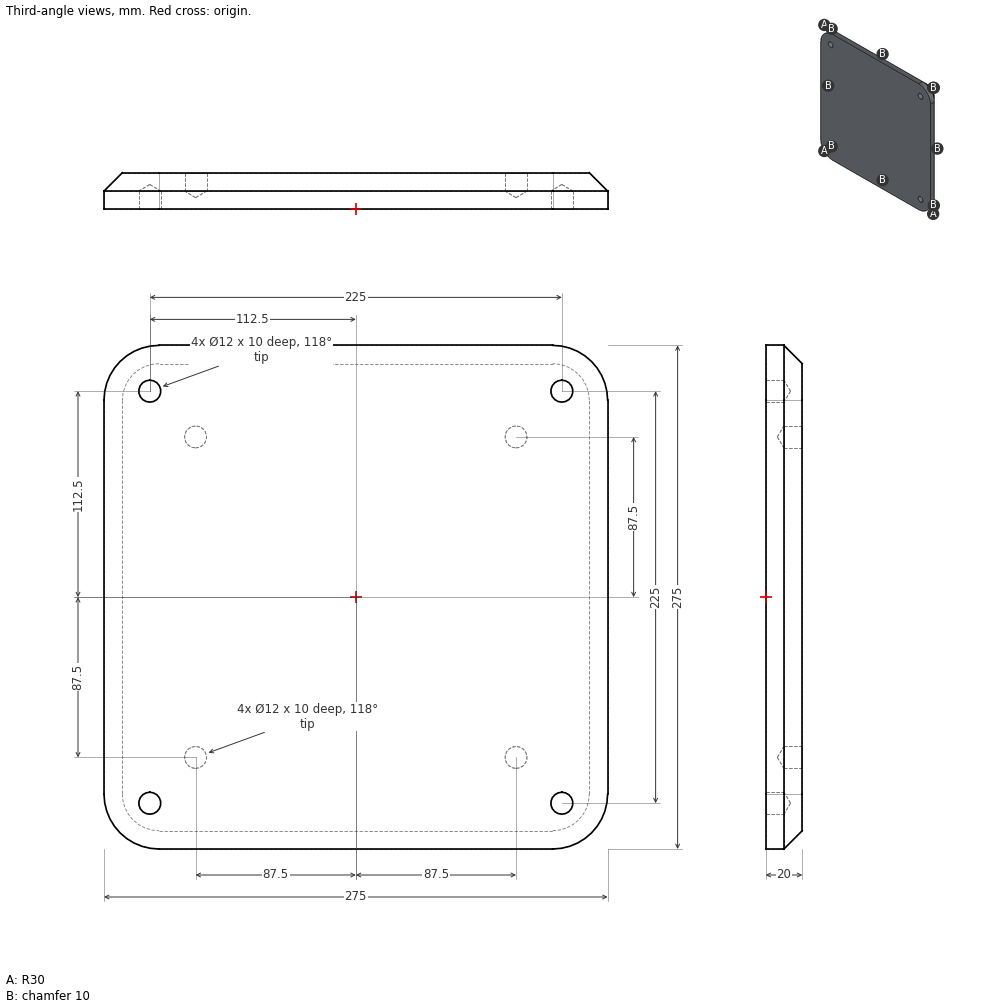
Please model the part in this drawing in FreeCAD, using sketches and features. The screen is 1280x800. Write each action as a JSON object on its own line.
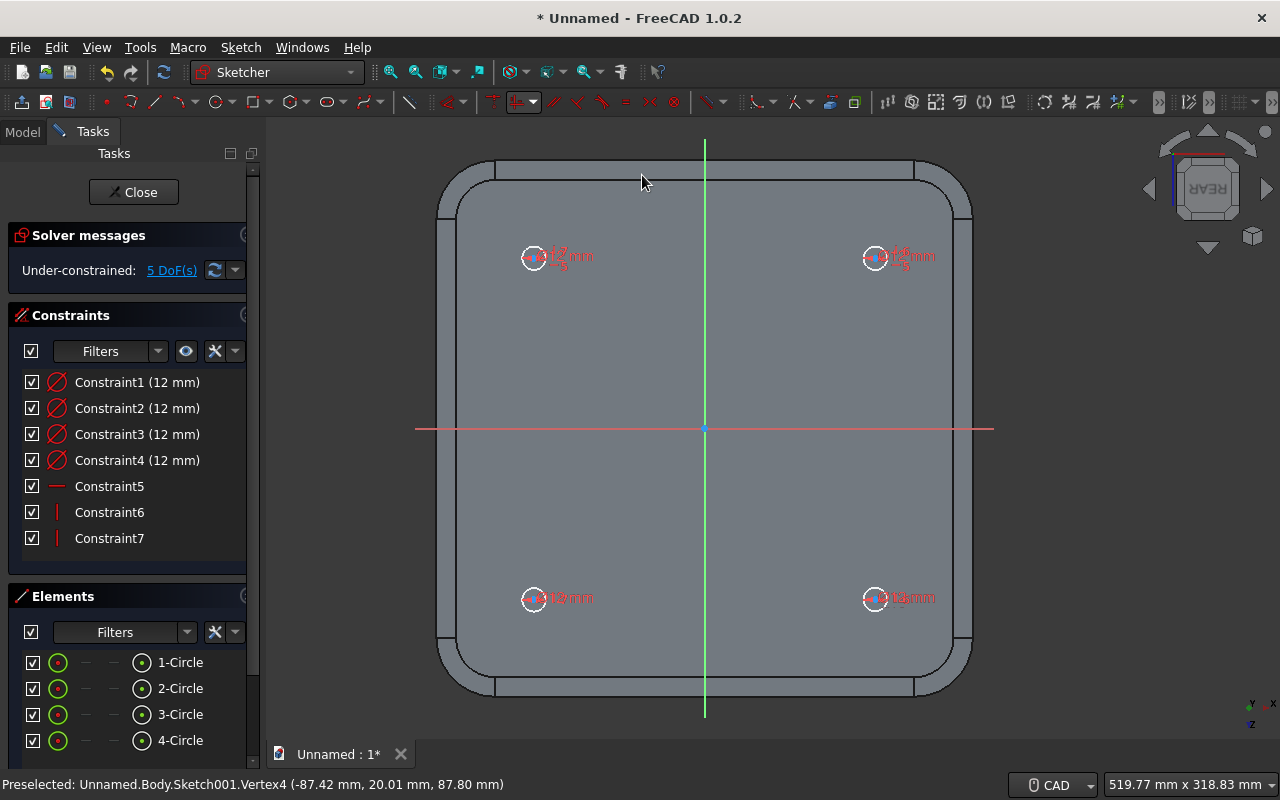
{"action": "left_click", "coordinate": [875, 600]}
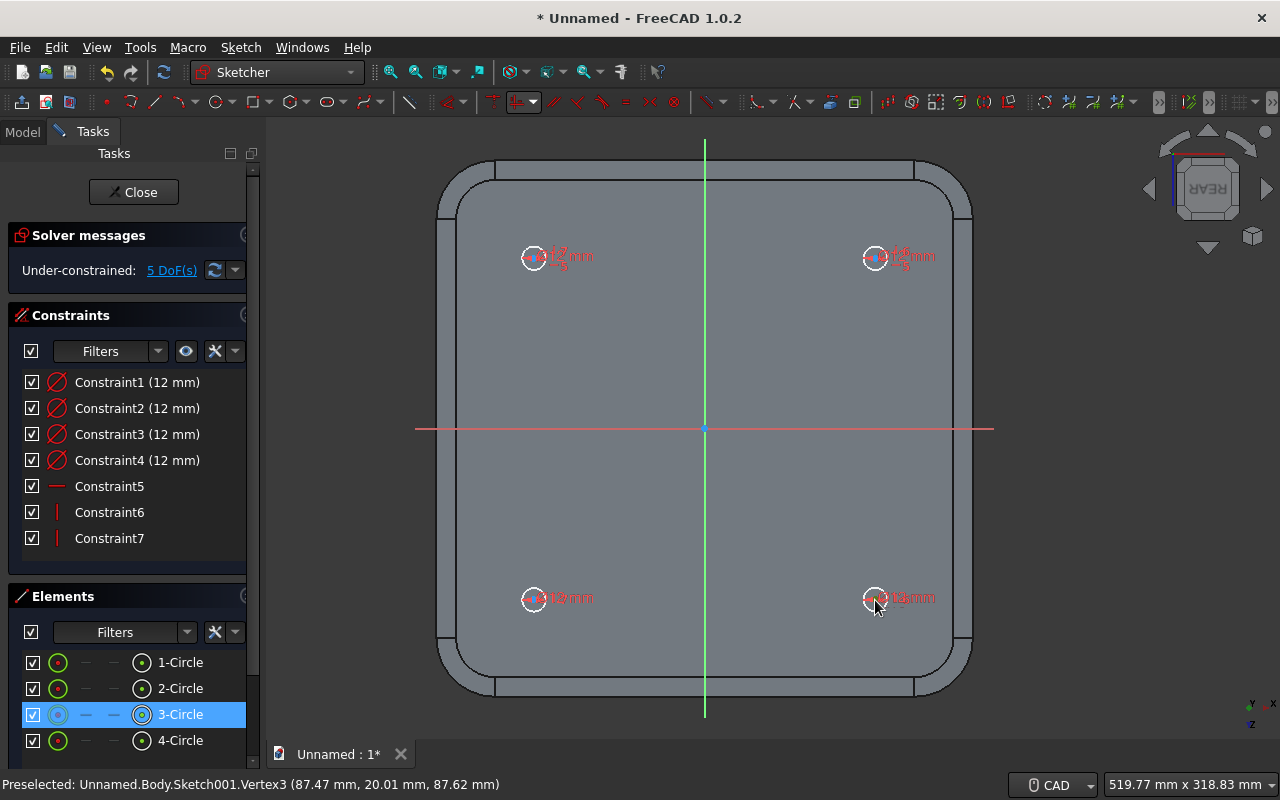
{"action": "left_click", "coordinate": [534, 600]}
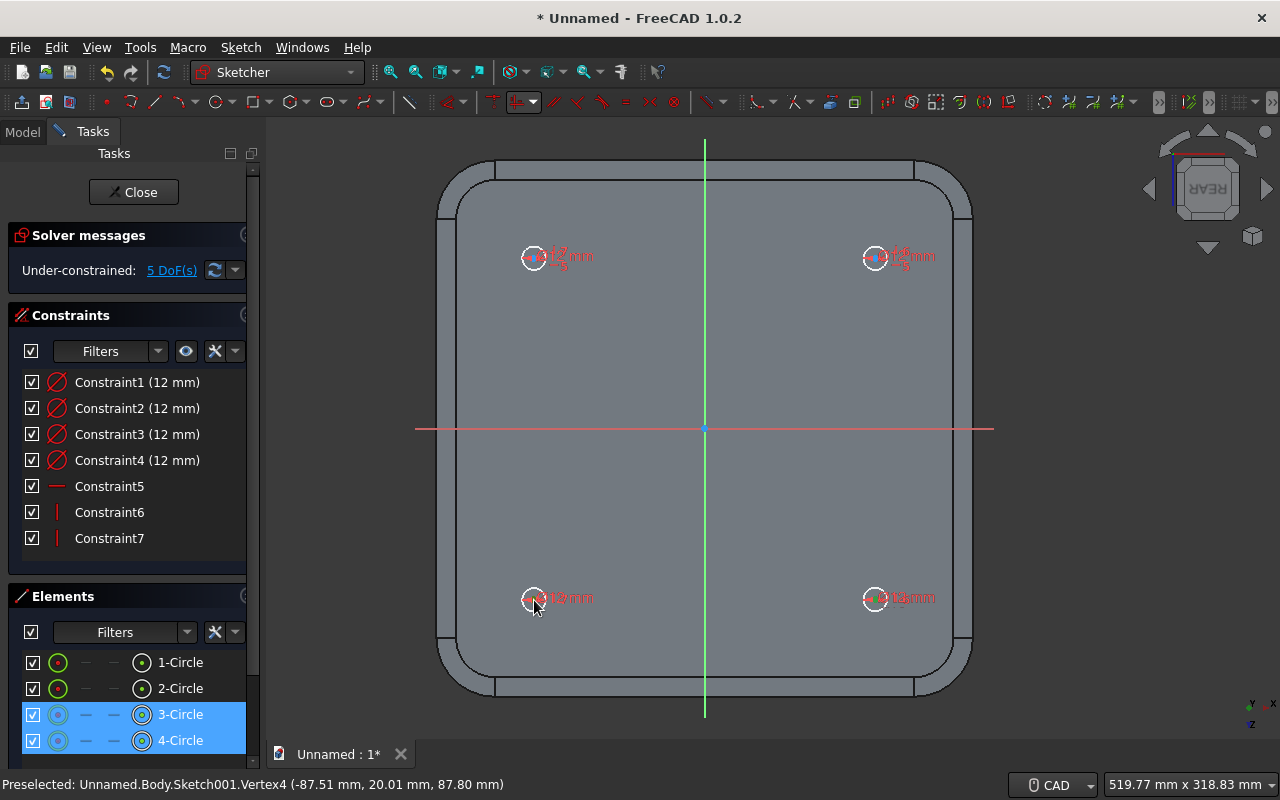
{"action": "key", "text": "h"}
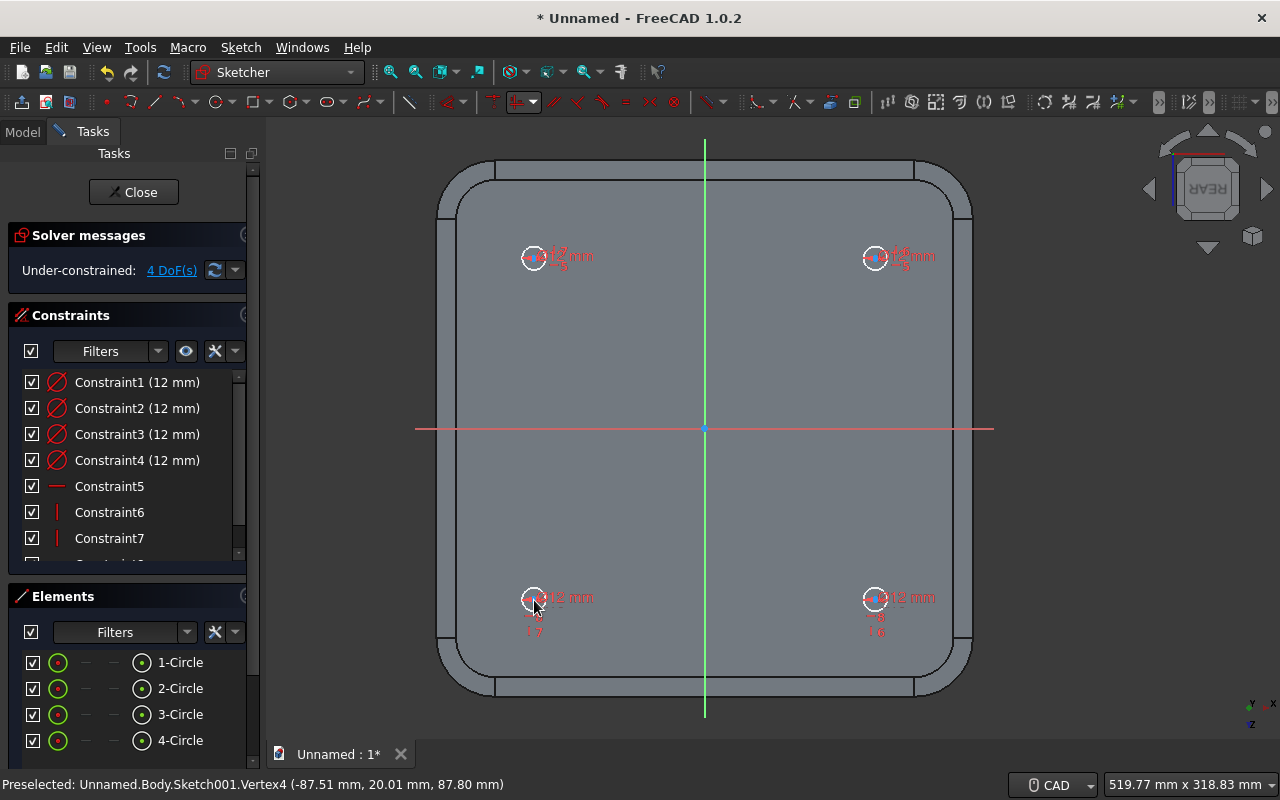
{"action": "key", "text": "d"}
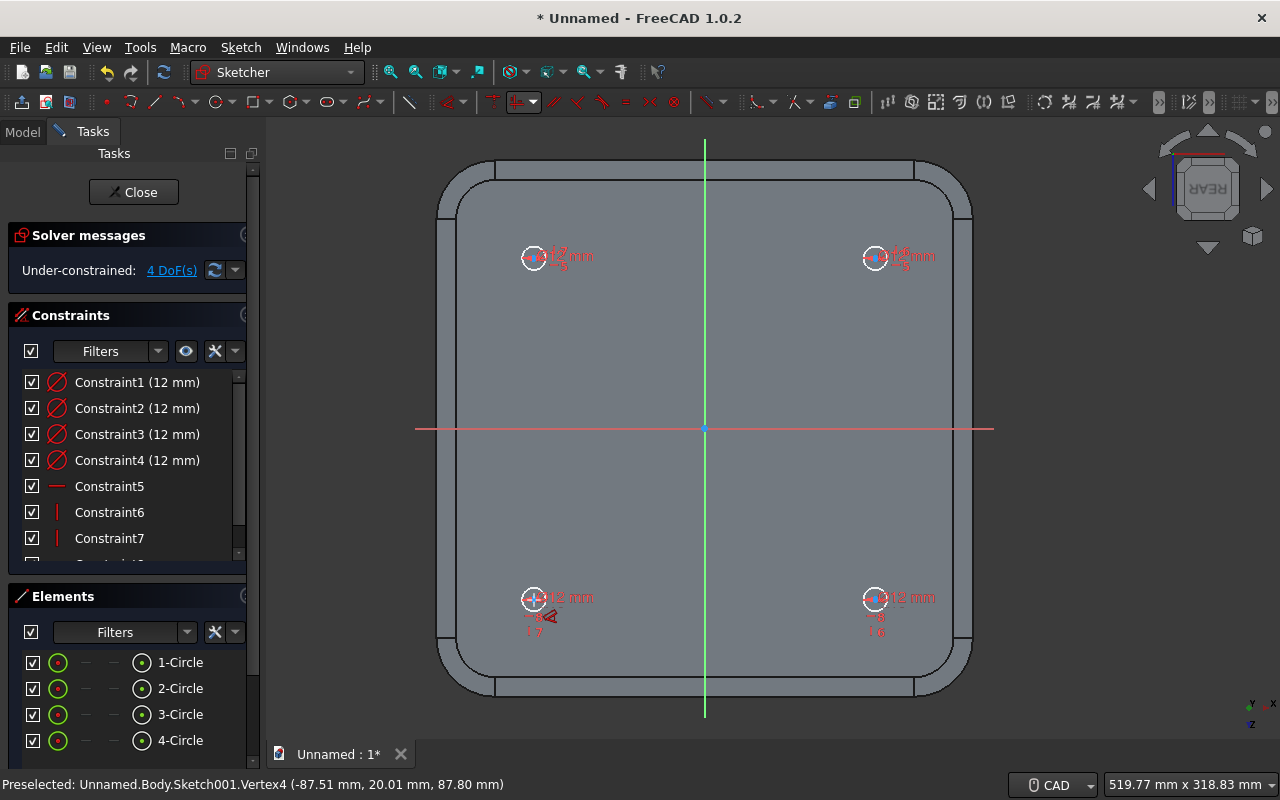
{"action": "left_click", "coordinate": [534, 258]}
{"action": "left_click", "coordinate": [619, 224]}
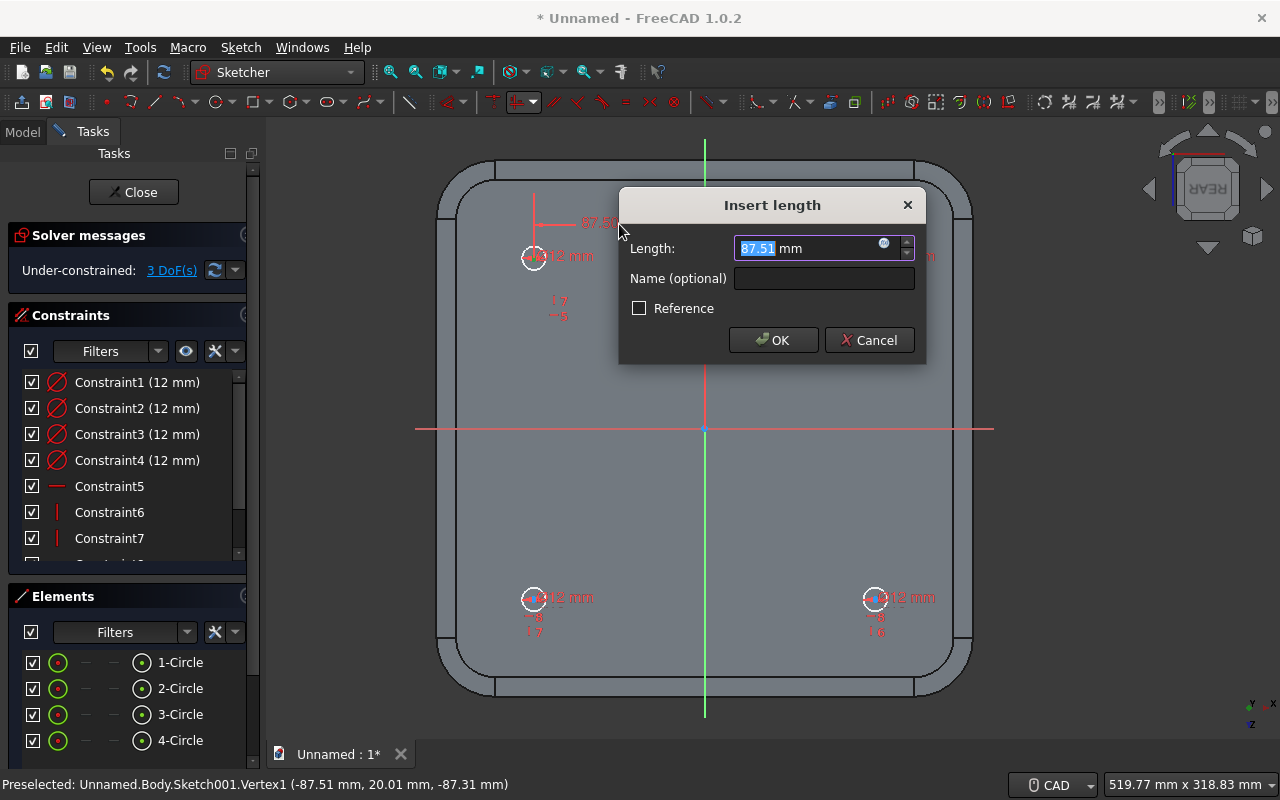
{"action": "type", "text": "87.5"}
{"action": "key", "text": "Return"}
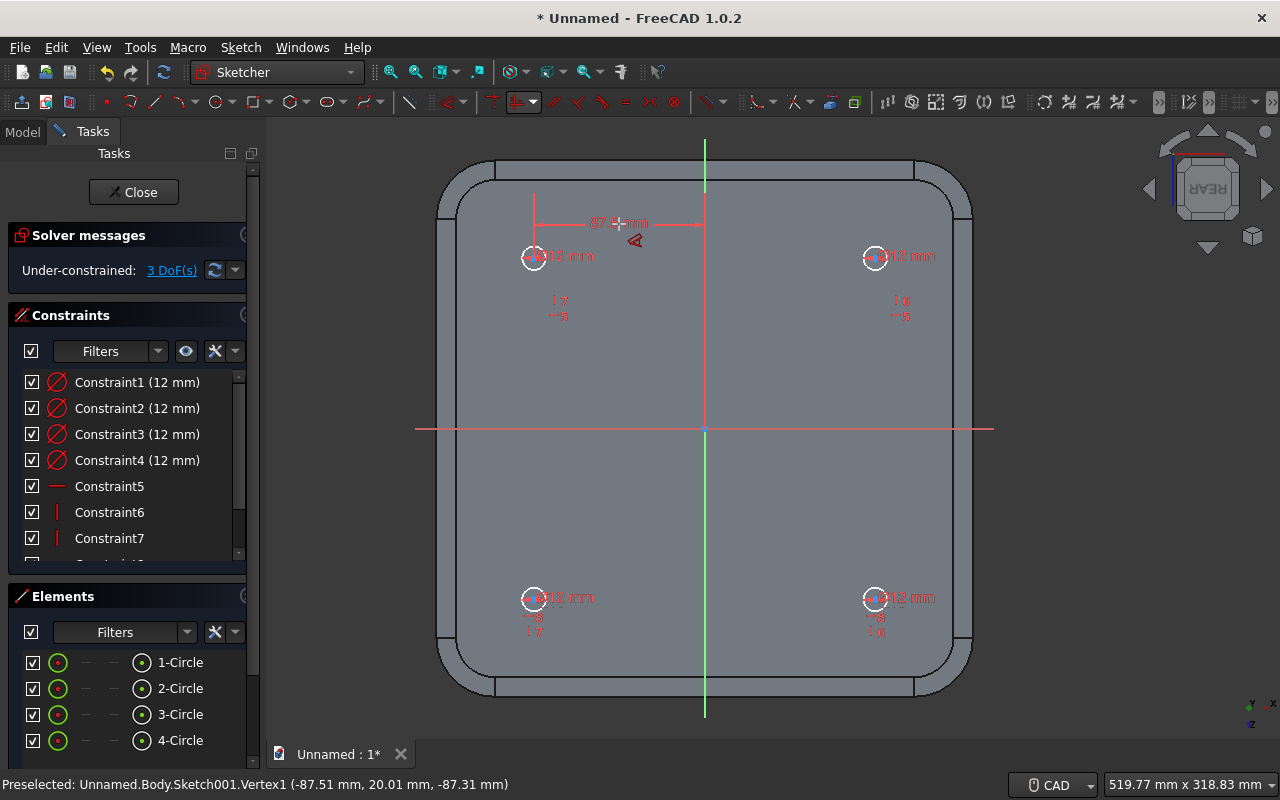
{"action": "left_click", "coordinate": [534, 258]}
{"action": "left_click", "coordinate": [500, 343]}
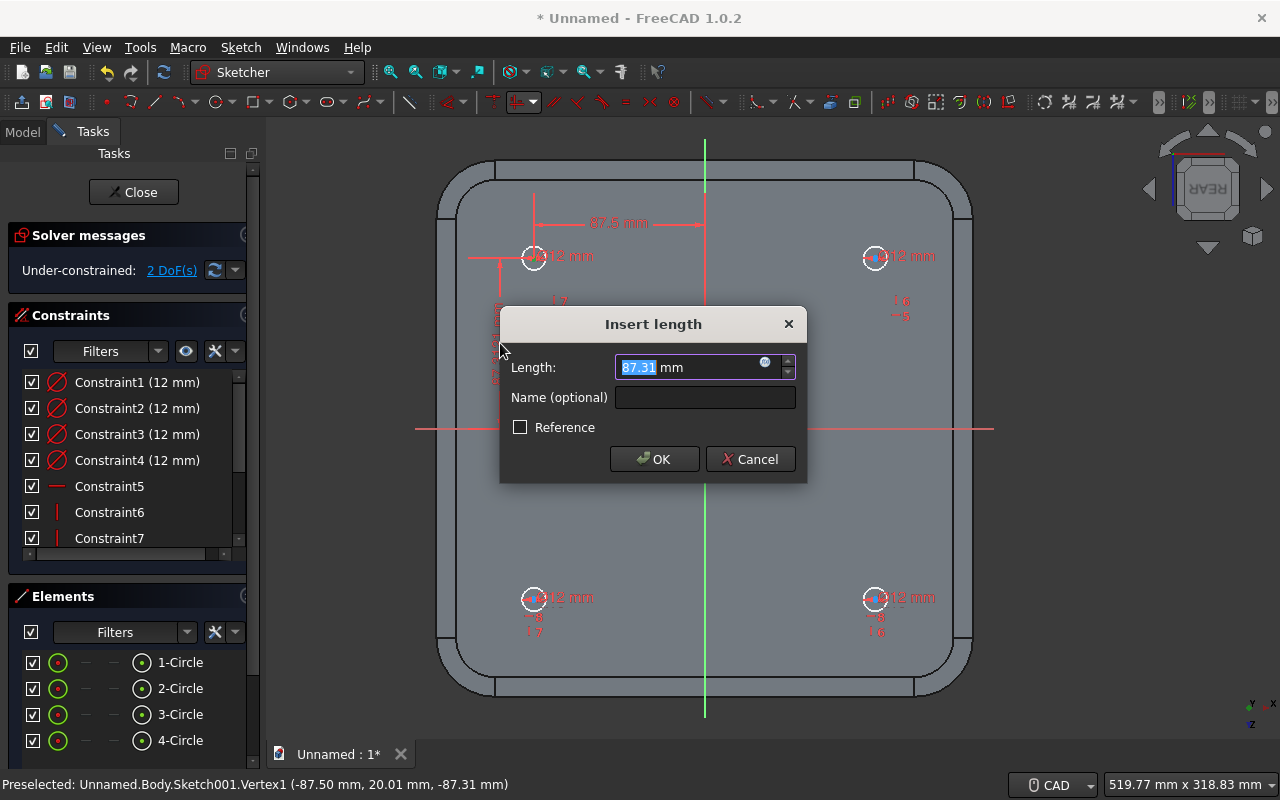
{"action": "type", "text": "87.5"}
{"action": "key", "text": "Return"}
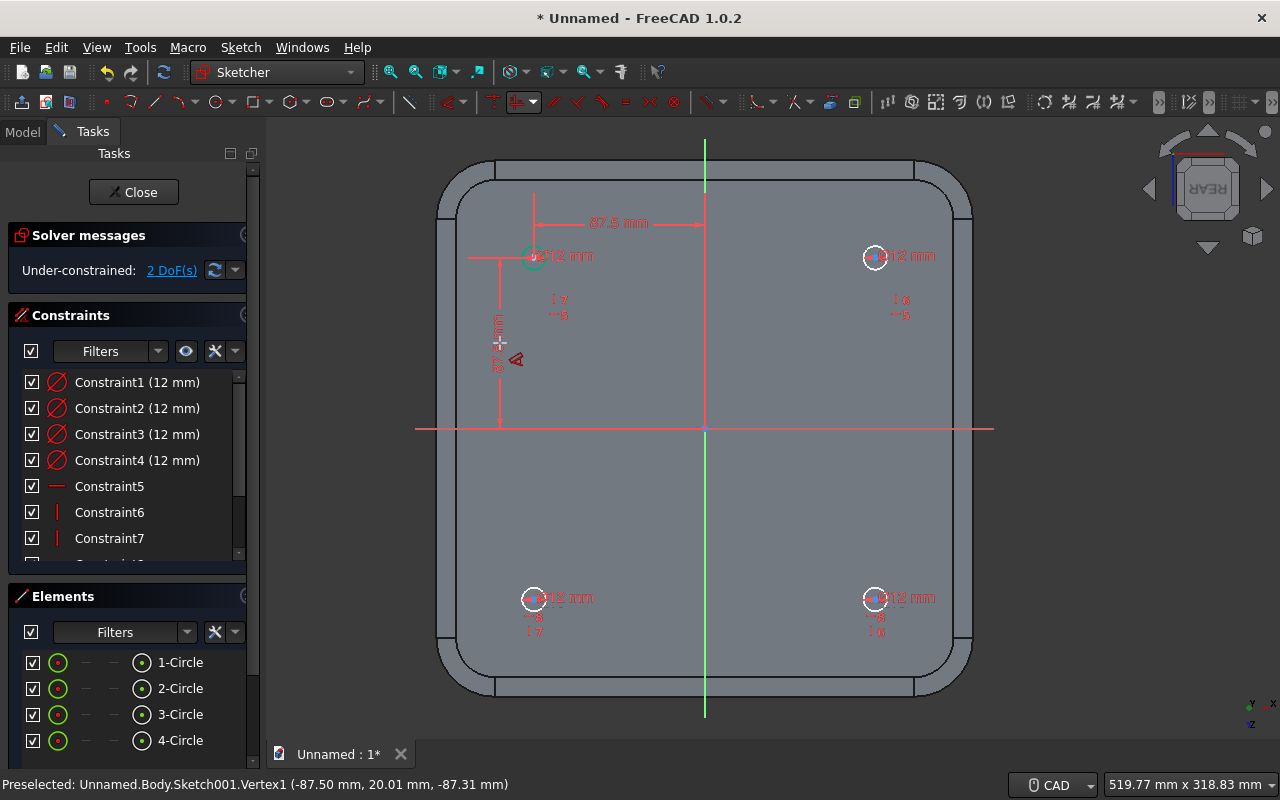
{"action": "left_click", "coordinate": [875, 258]}
{"action": "left_click", "coordinate": [790, 224]}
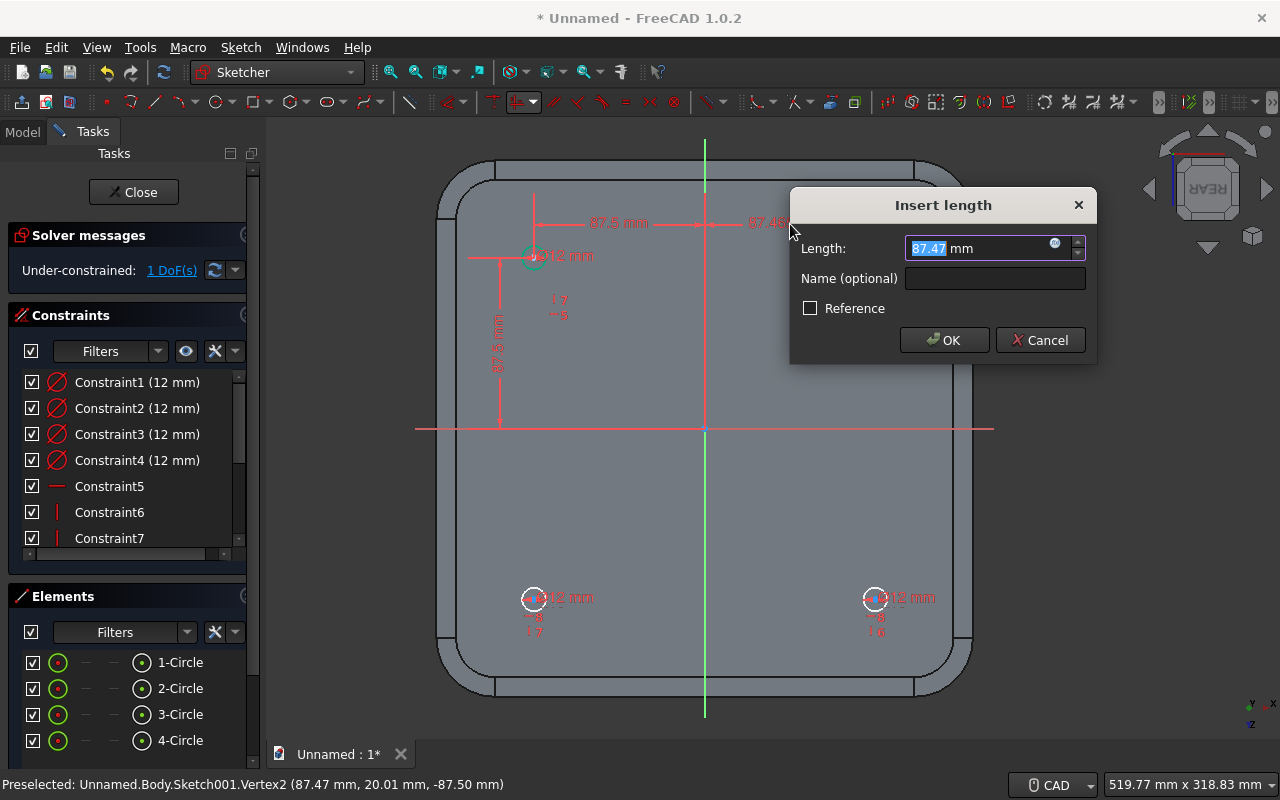
{"action": "type", "text": "87.5"}
{"action": "key", "text": "Return"}